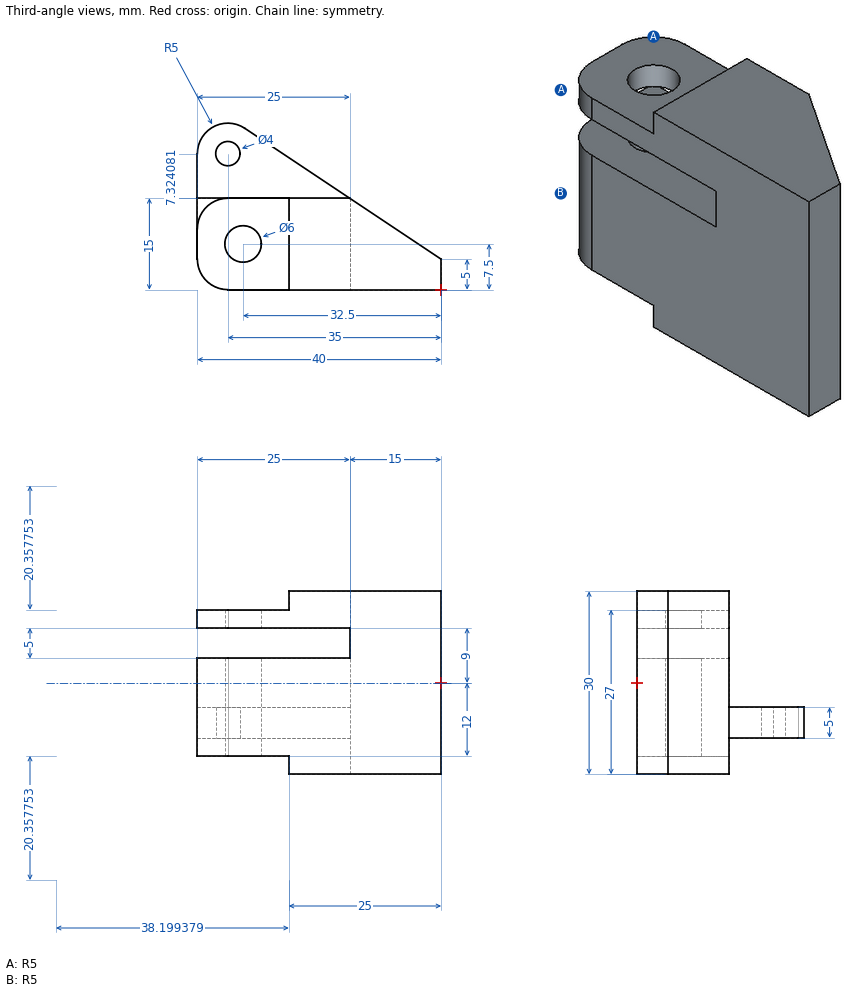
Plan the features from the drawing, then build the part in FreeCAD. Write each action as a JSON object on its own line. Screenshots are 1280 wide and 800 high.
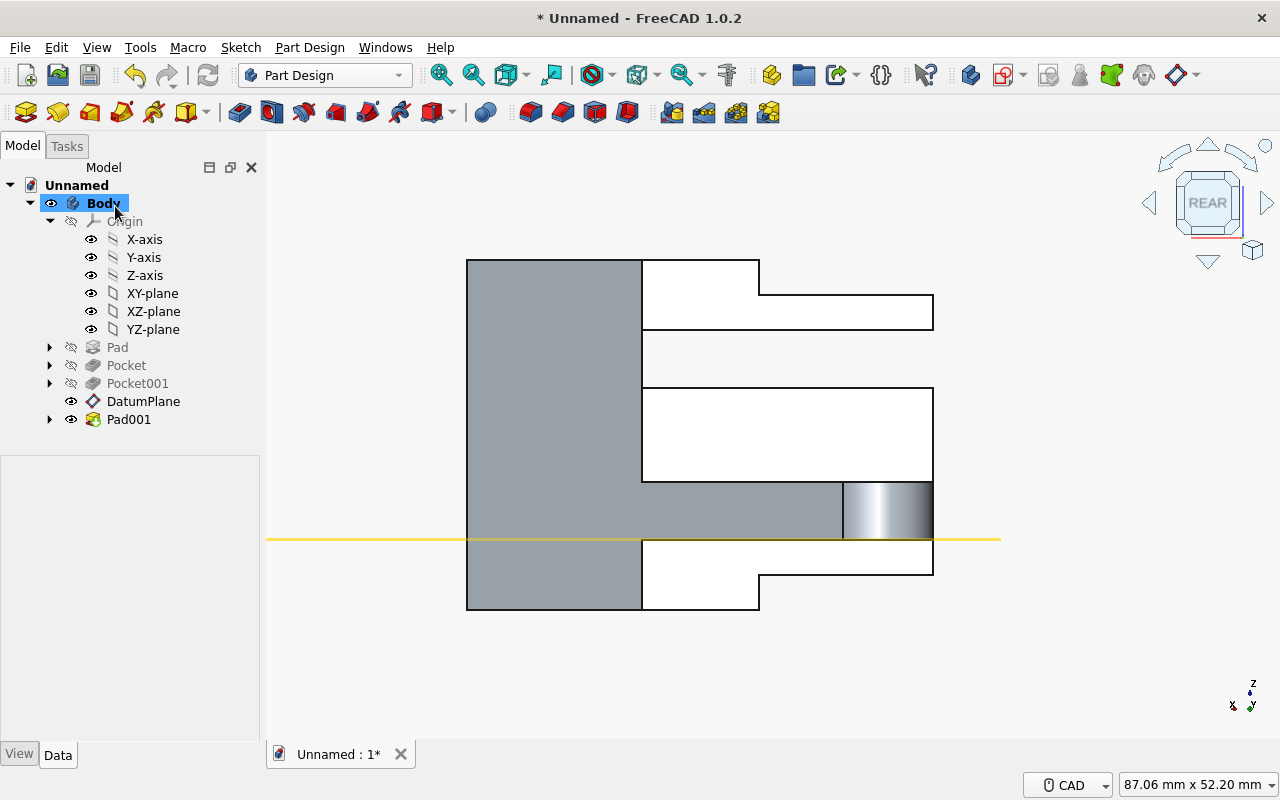
{"action": "left_click", "coordinate": [116, 401]}
{"action": "key", "text": "space"}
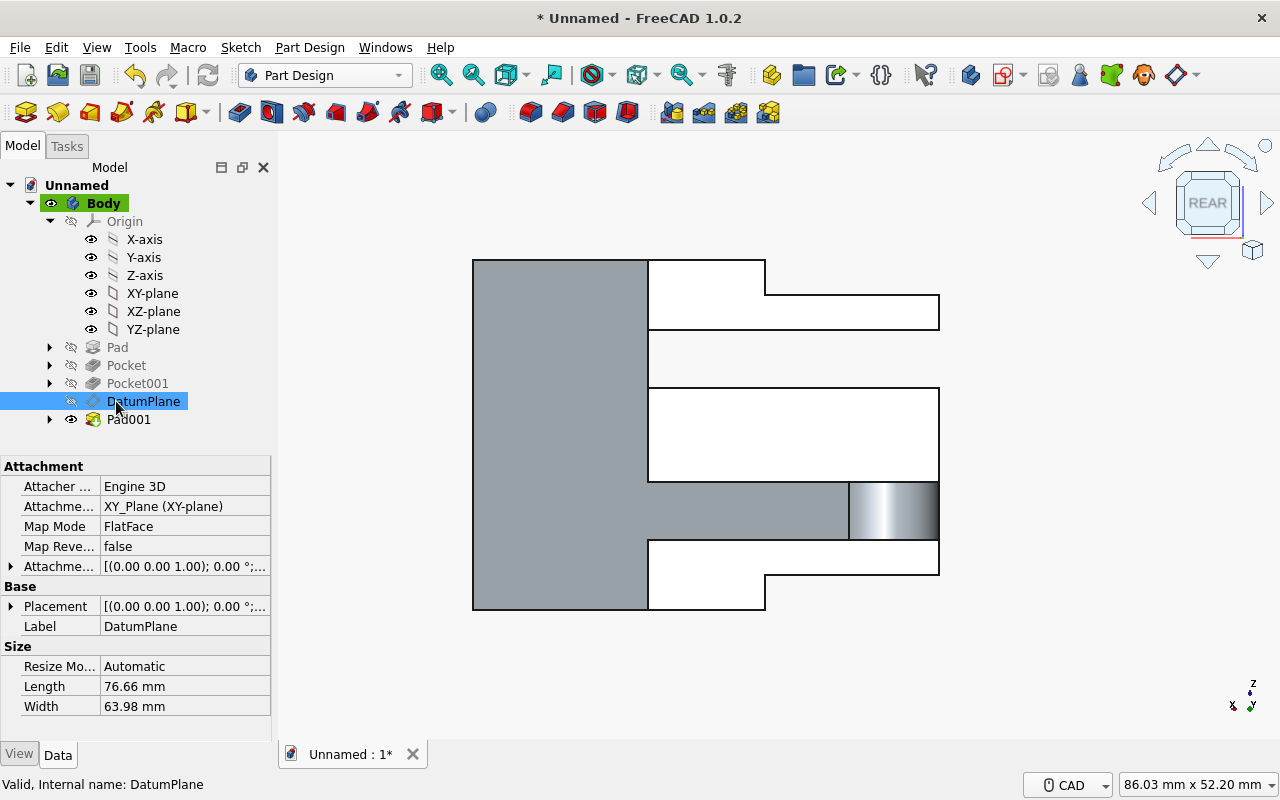
{"action": "key", "text": "0"}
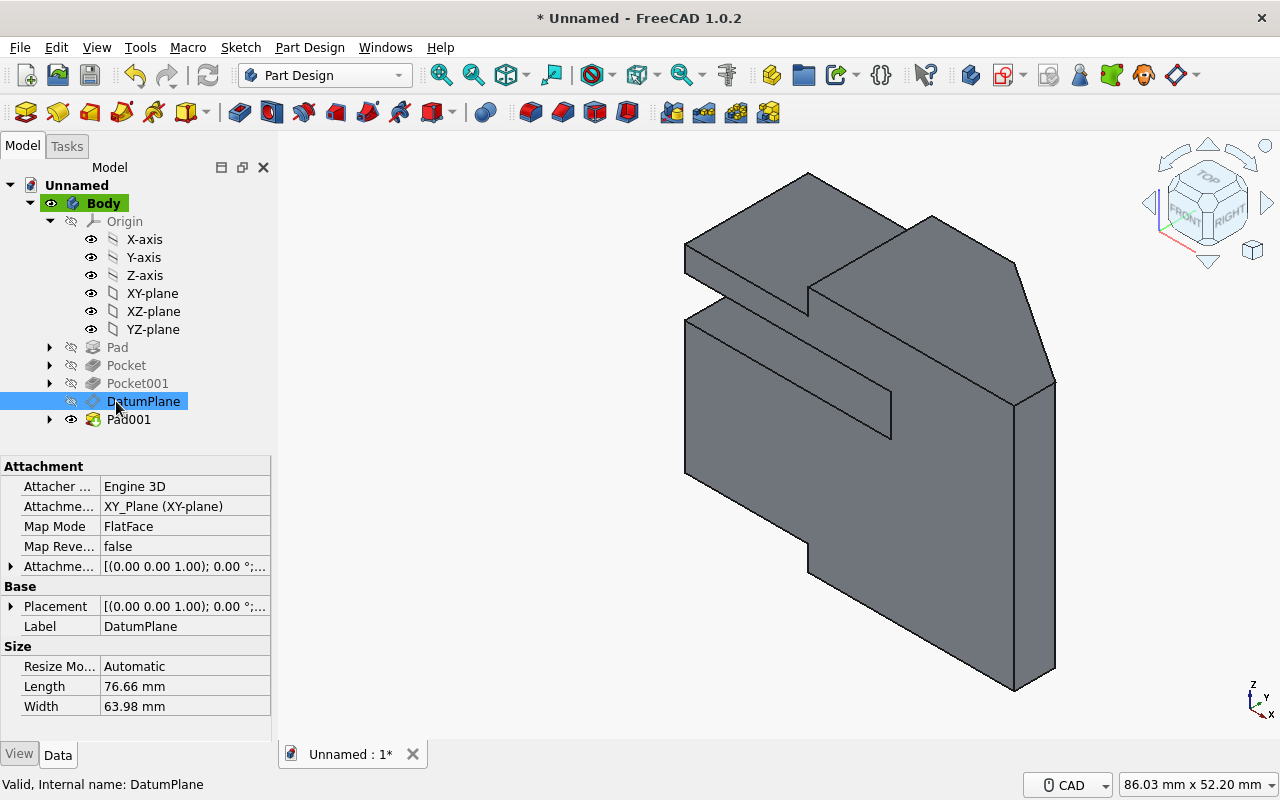
{"action": "key", "text": "v f"}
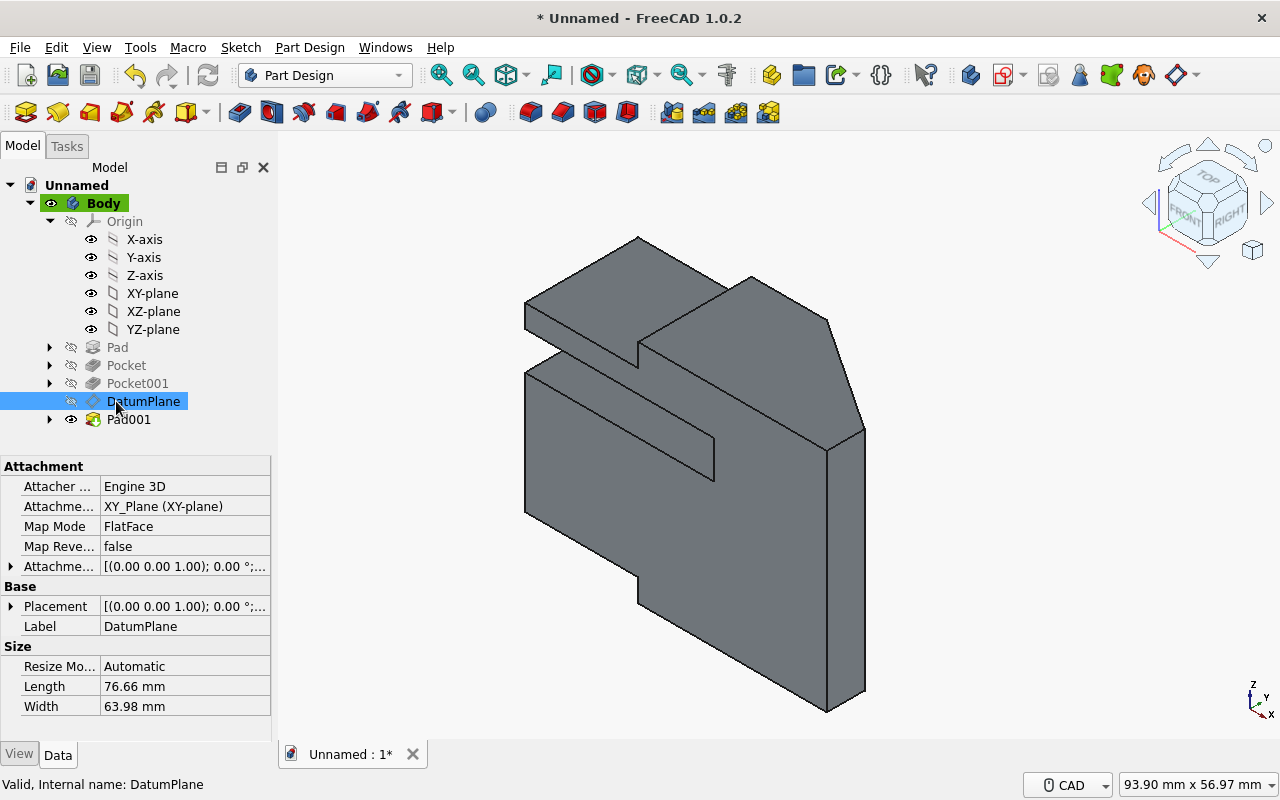
{"action": "left_click", "coordinate": [638, 302]}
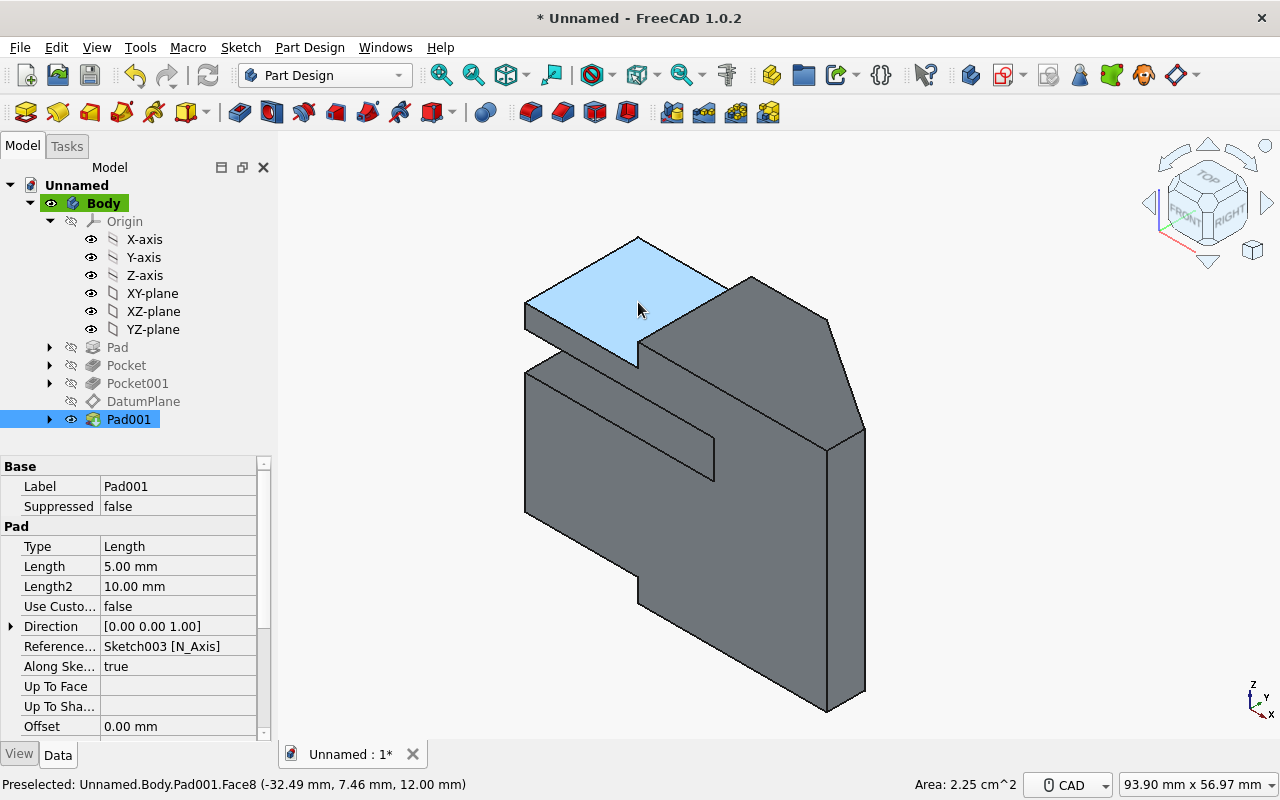
{"action": "left_click", "coordinate": [1004, 76]}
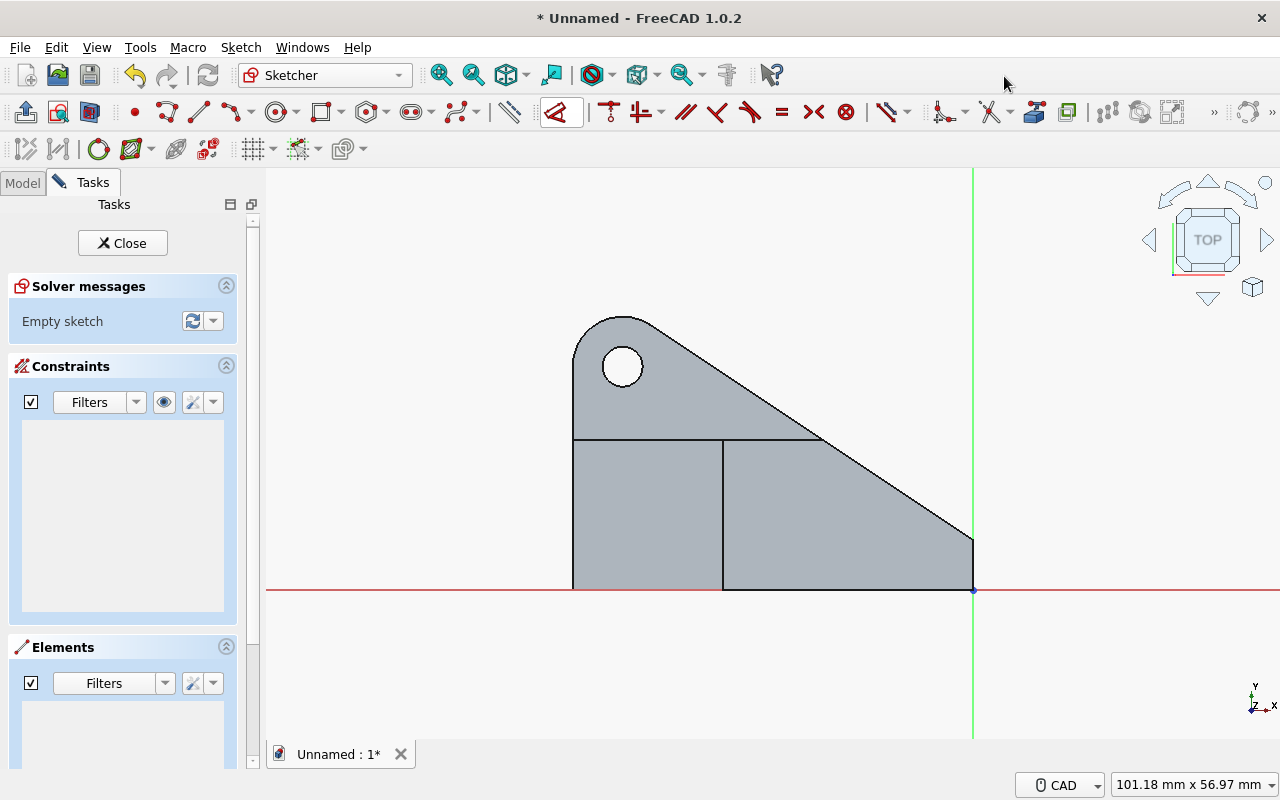
{"action": "left_click", "coordinate": [90, 112]}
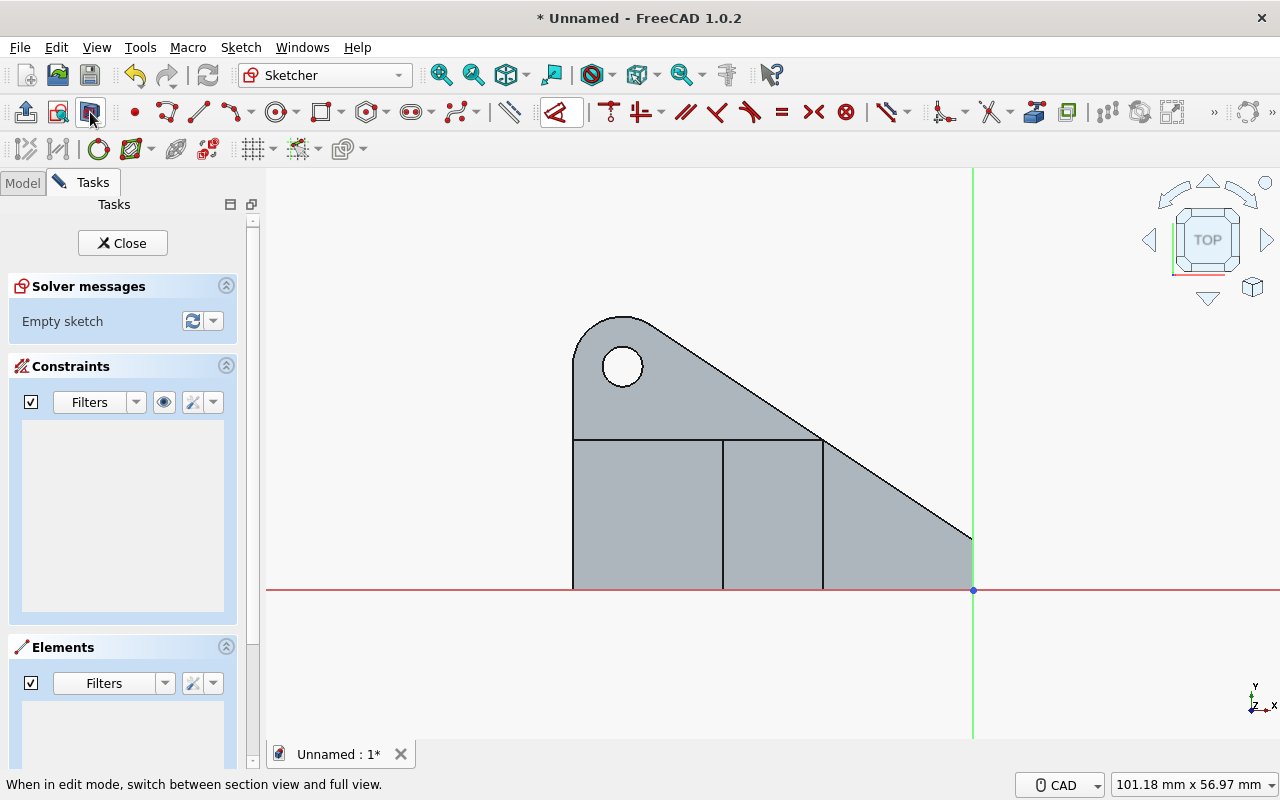
{"action": "scroll", "coordinate": [636, 527], "scroll_direction": "up", "scroll_amount": 9}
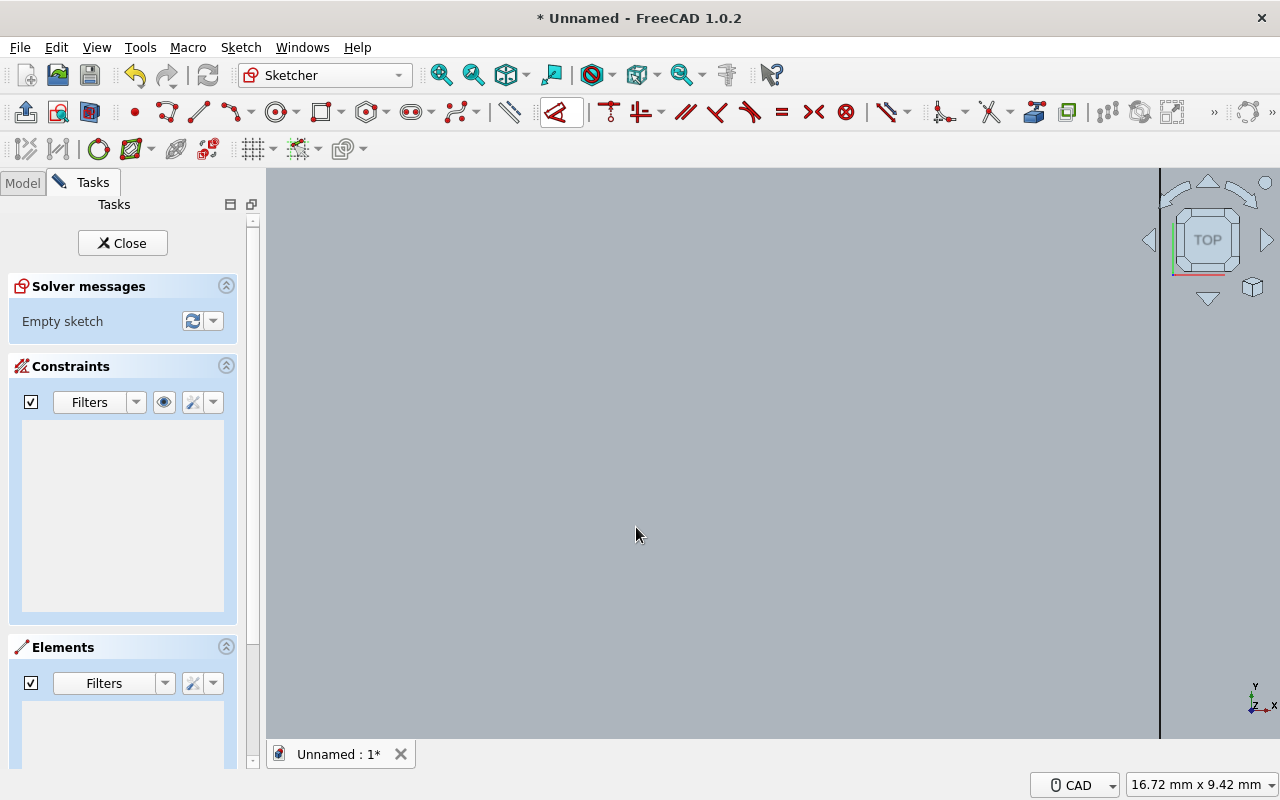
{"action": "key", "text": "g c"}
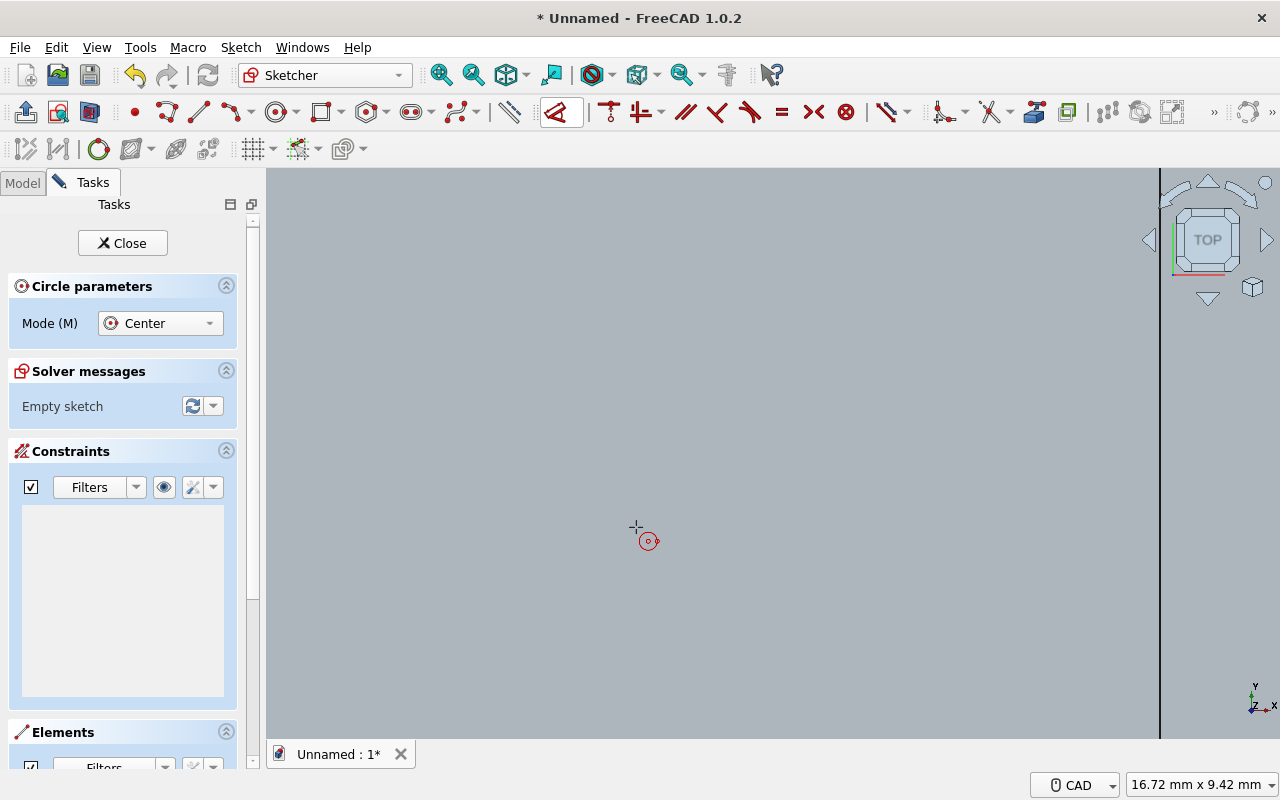
{"action": "left_click", "coordinate": [705, 453]}
{"action": "mouse_move", "coordinate": [834, 324]}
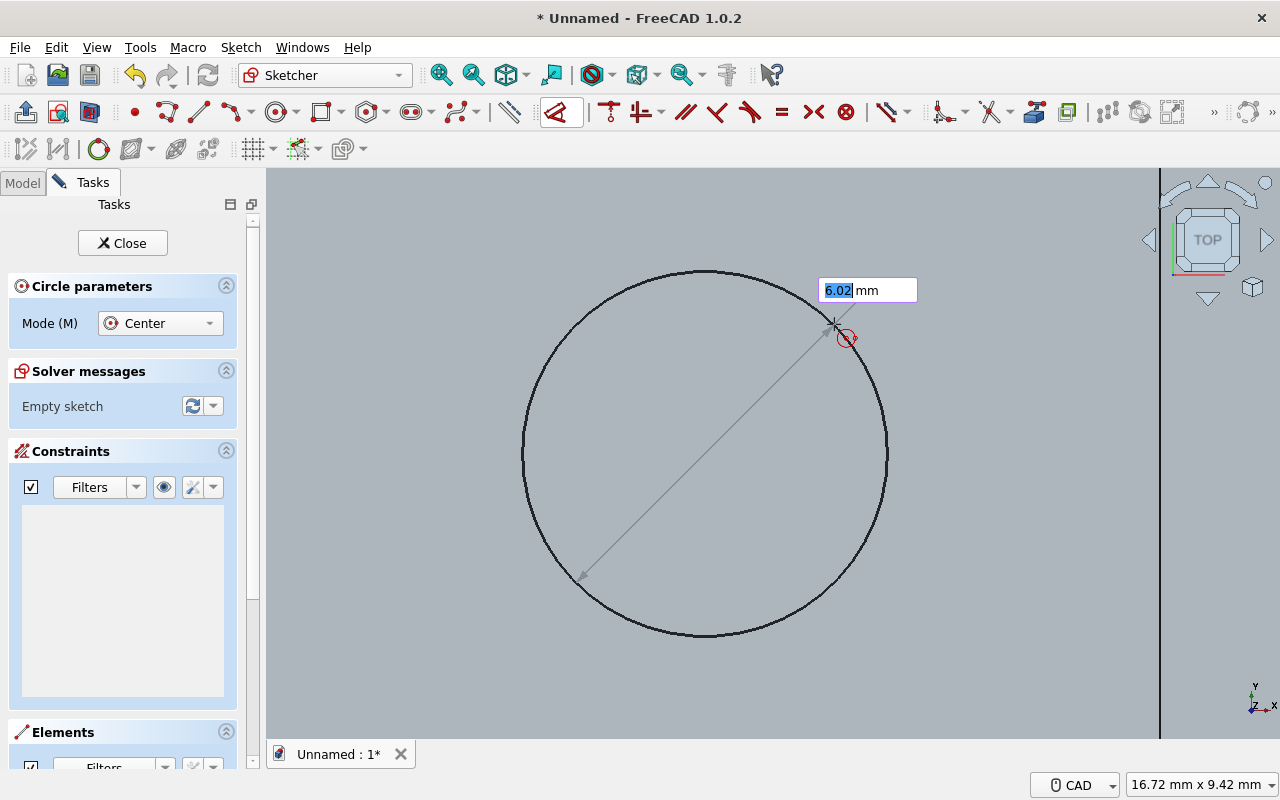
{"action": "type", "text": "6"}
{"action": "key", "text": "Return"}
{"action": "key", "text": "Escape"}